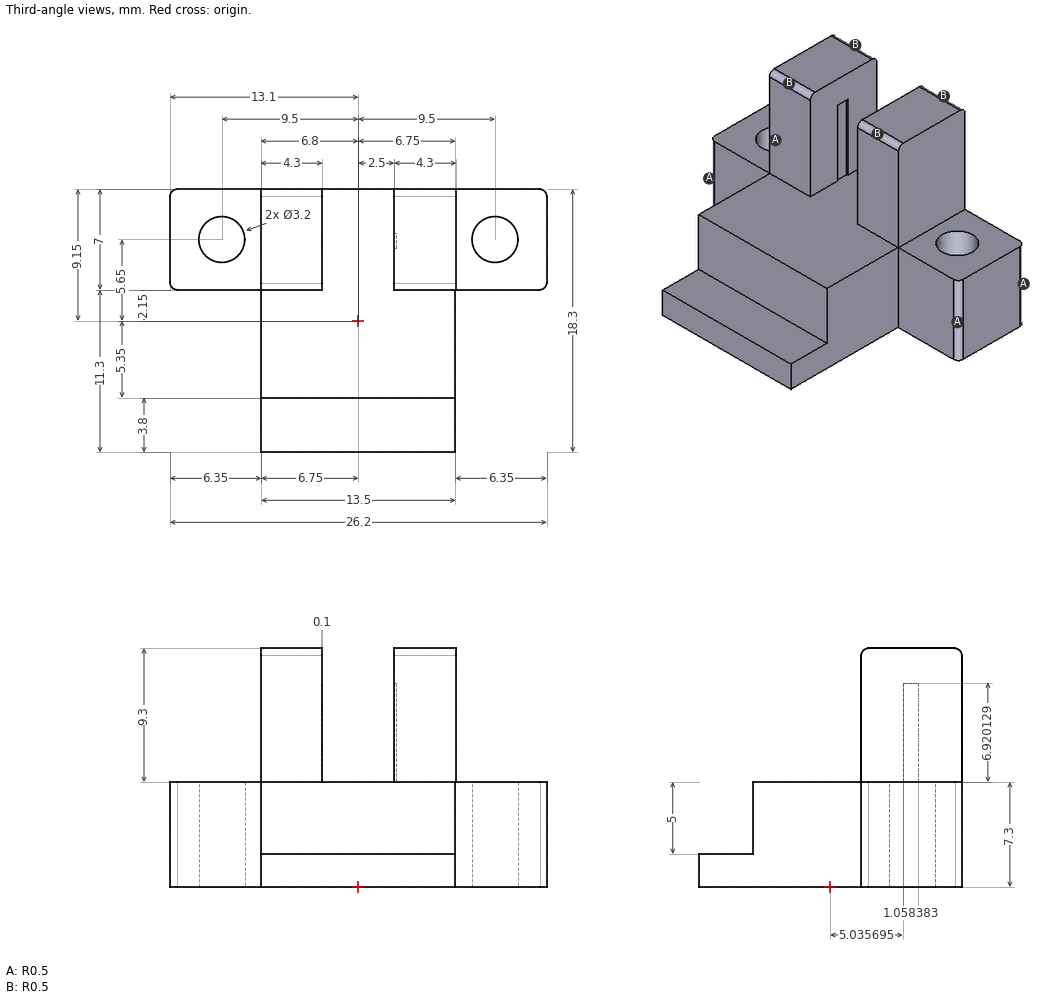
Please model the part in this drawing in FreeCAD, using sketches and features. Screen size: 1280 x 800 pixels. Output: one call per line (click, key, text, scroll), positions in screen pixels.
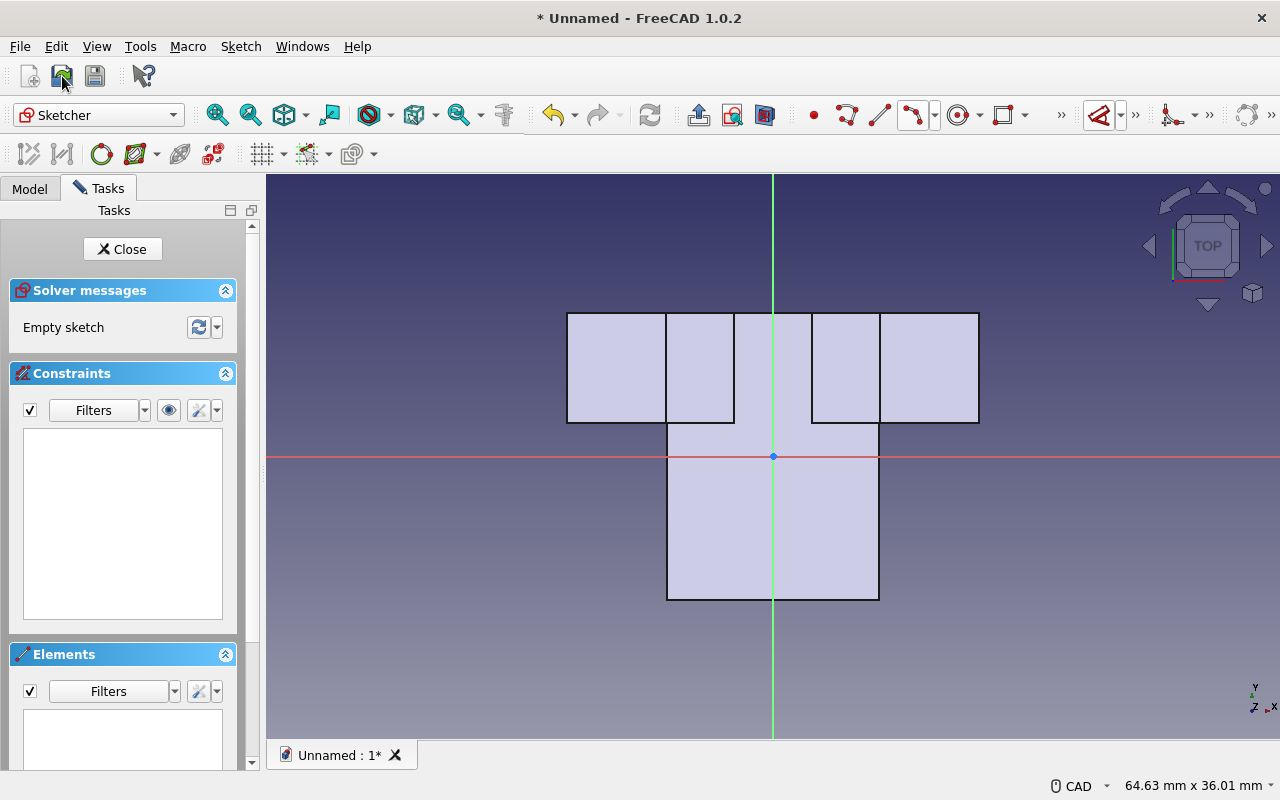
key(q)
key(s)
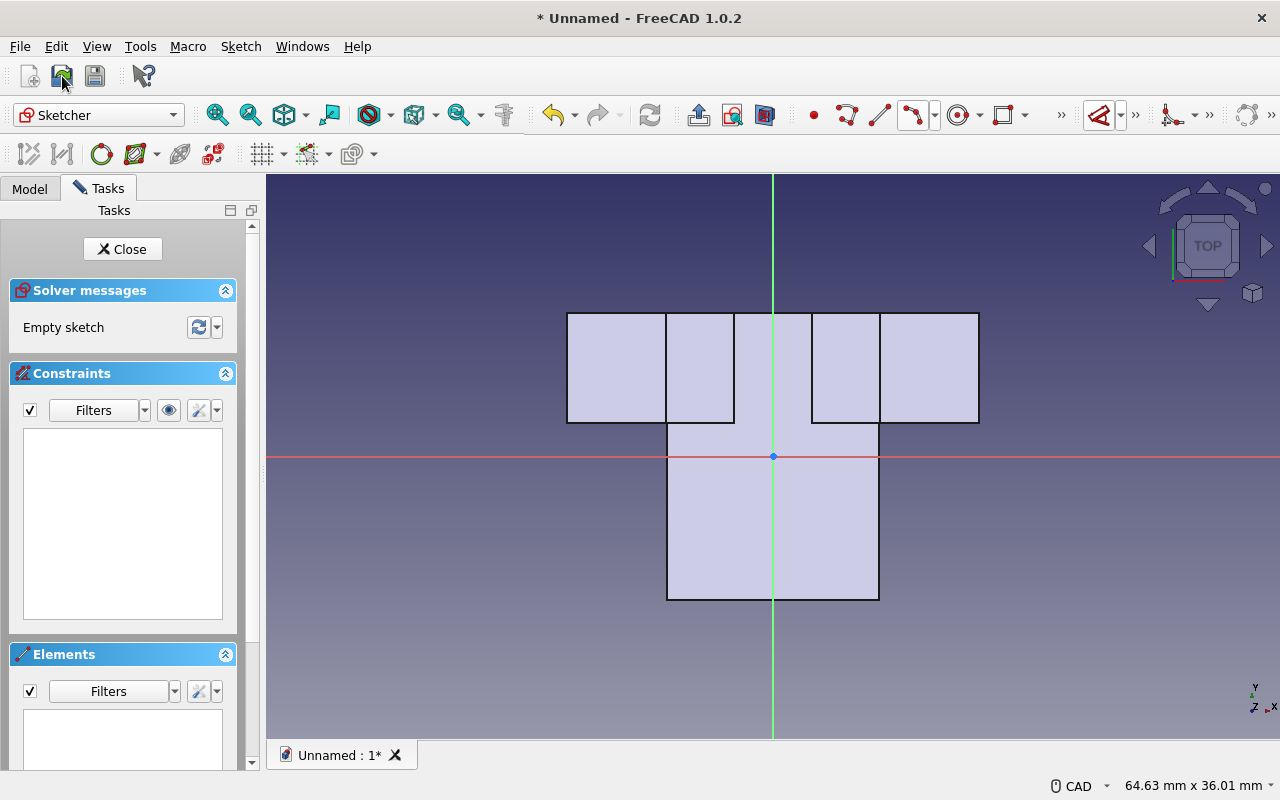
scroll(813, 570, up, 5)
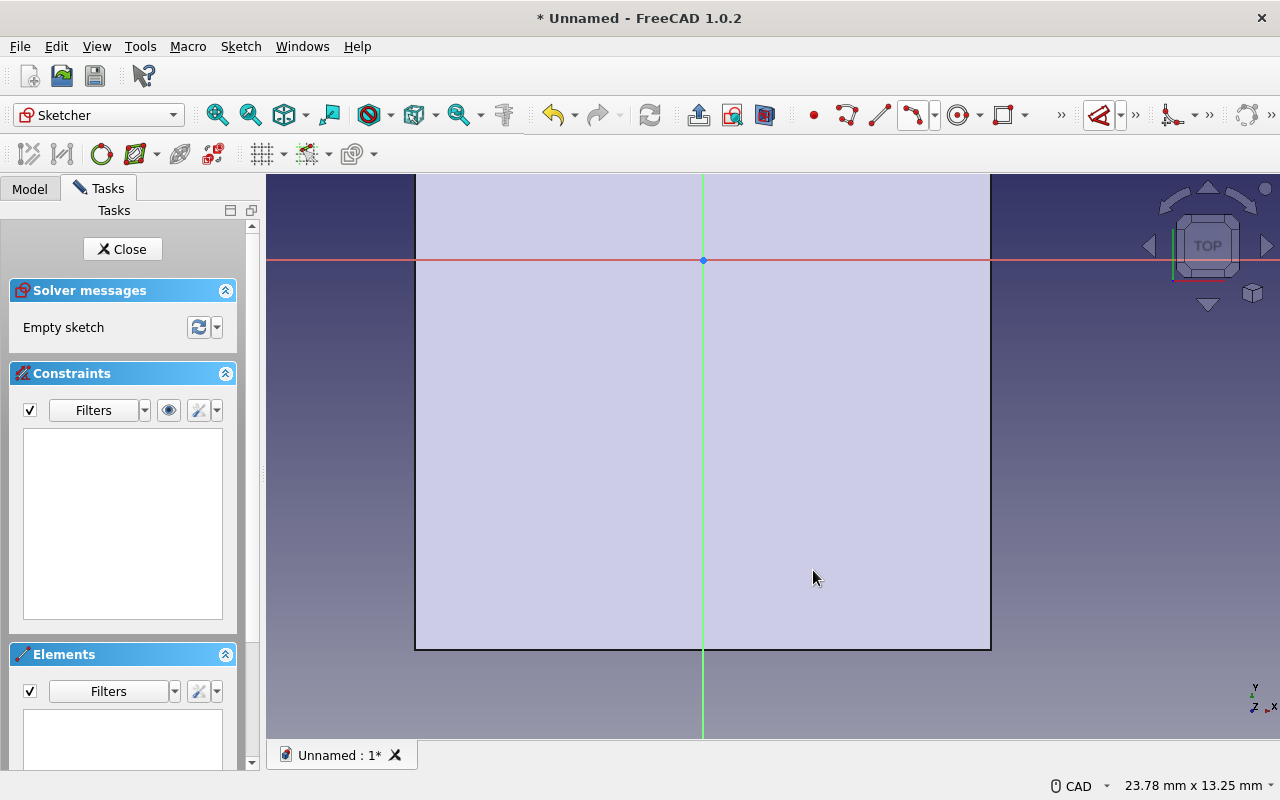
click(1002, 116)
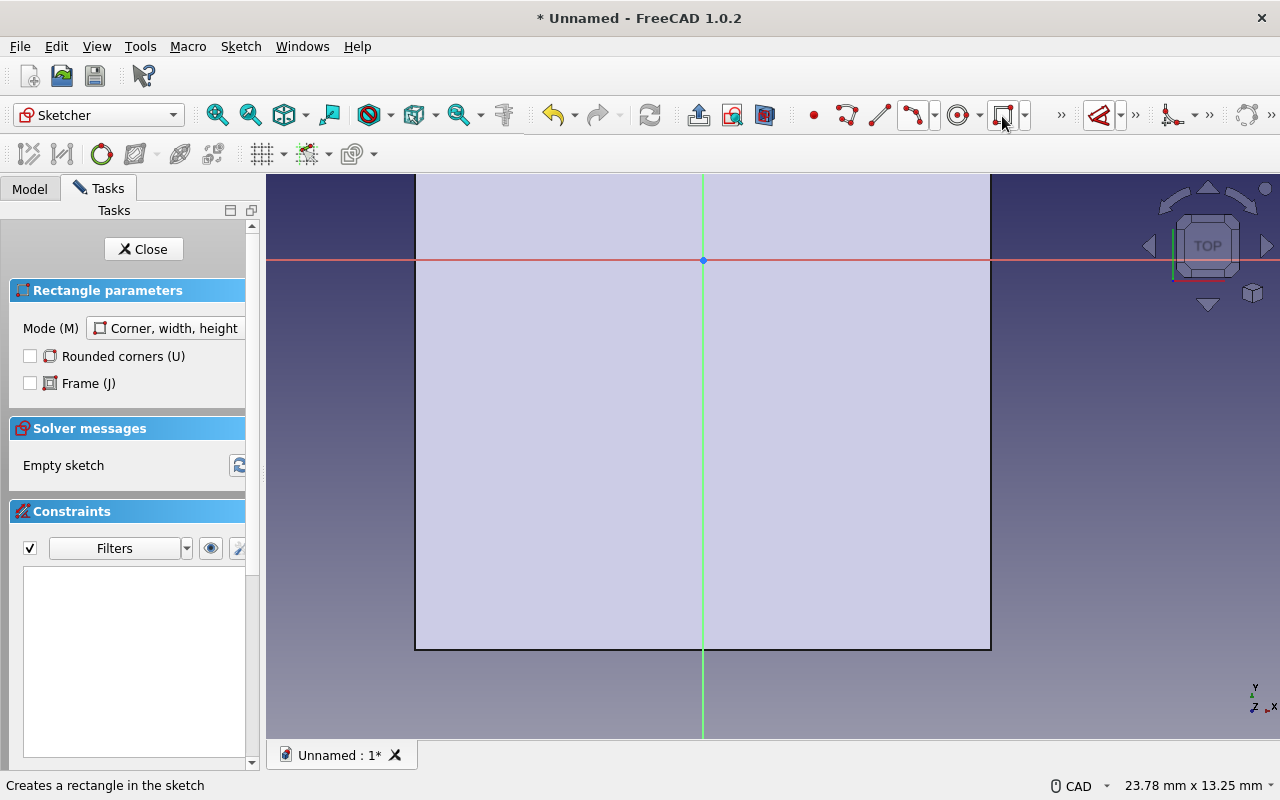
click(415, 488)
click(991, 650)
key(Escape)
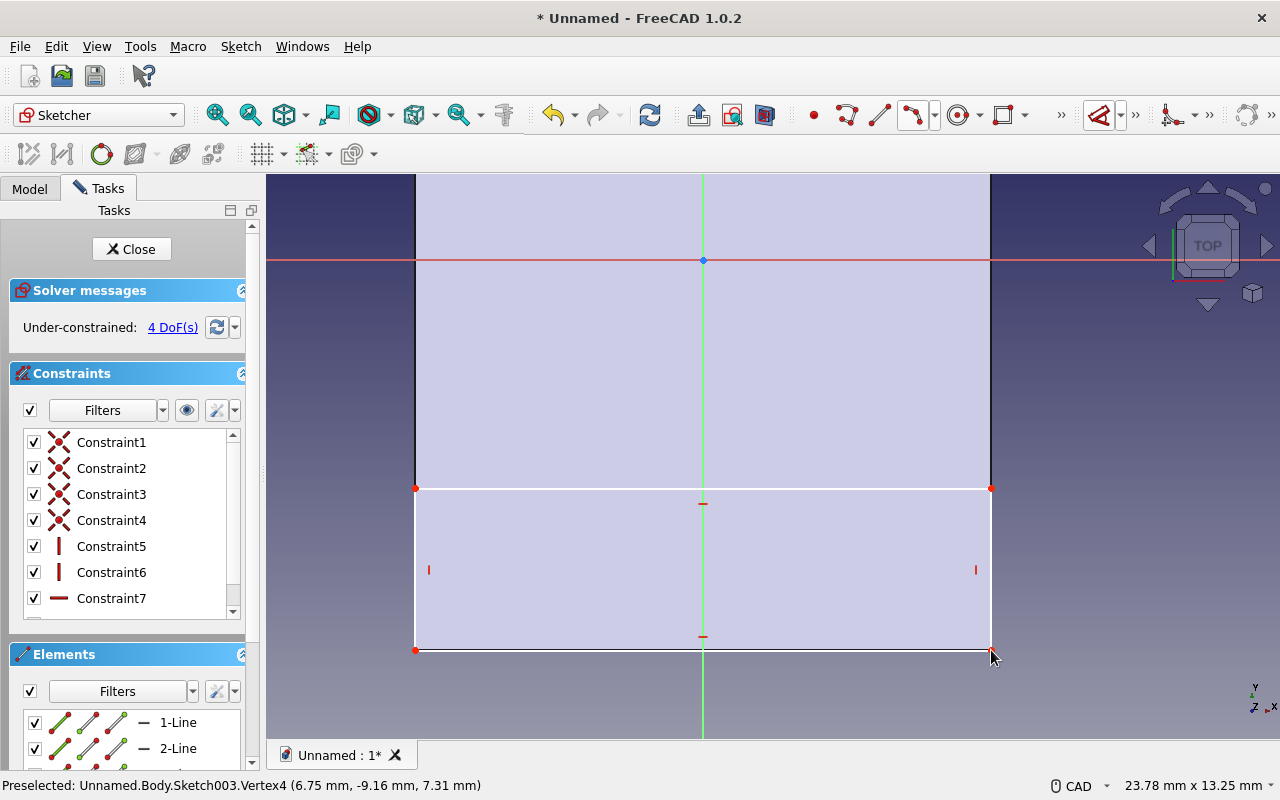
click(415, 538)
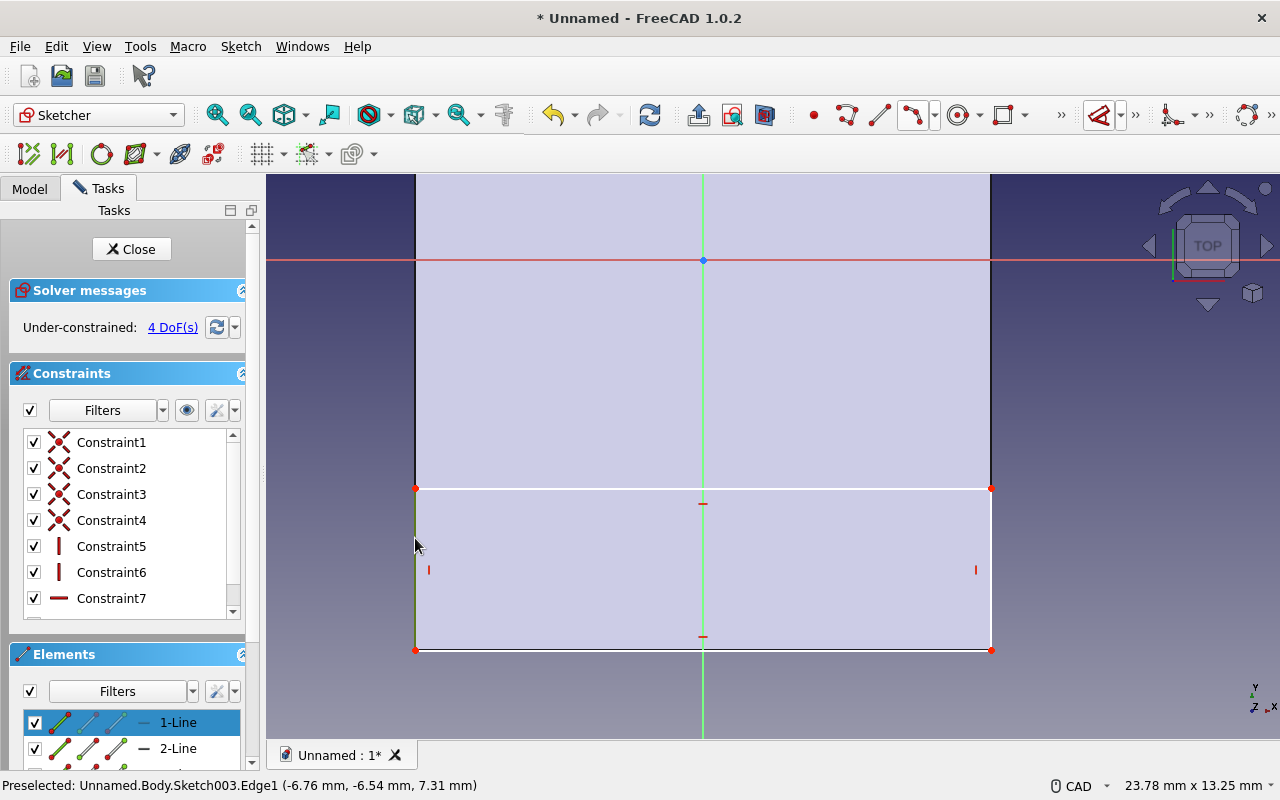
key(i)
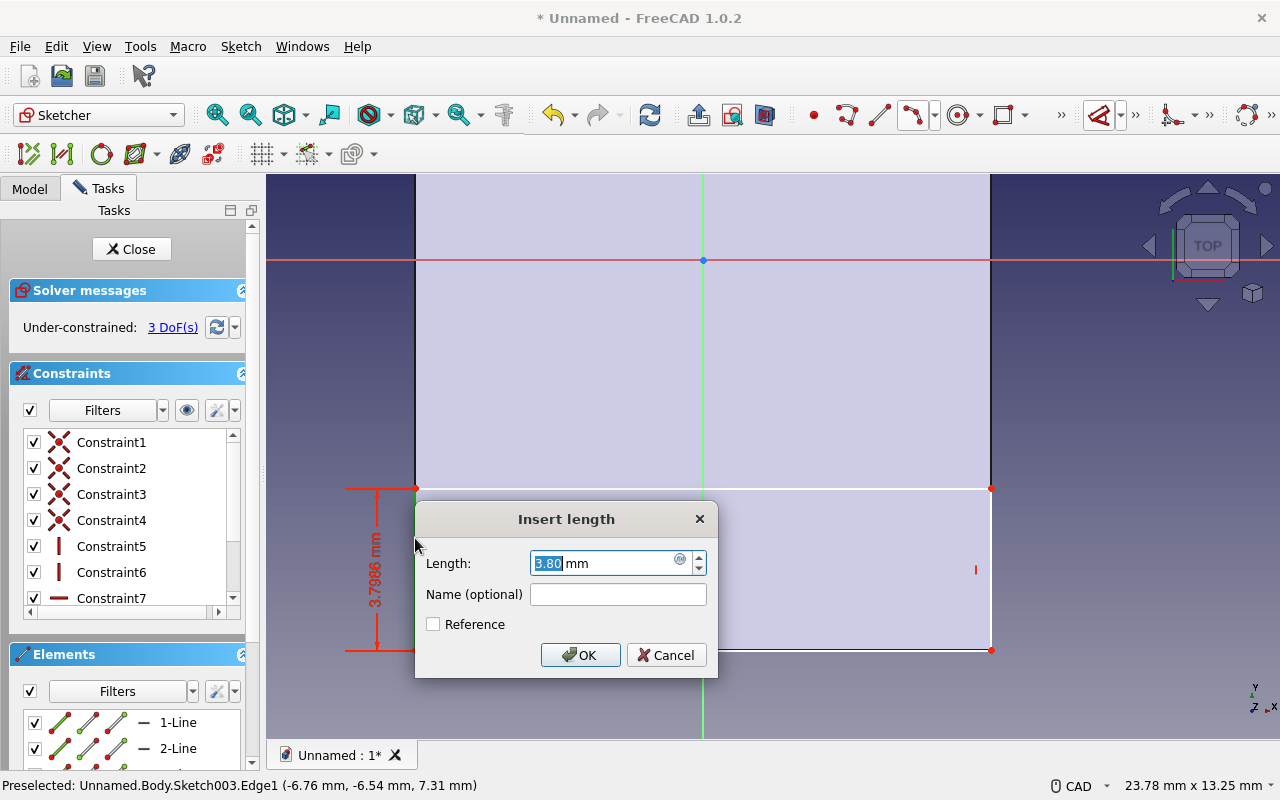
text(3.8)
key(Return)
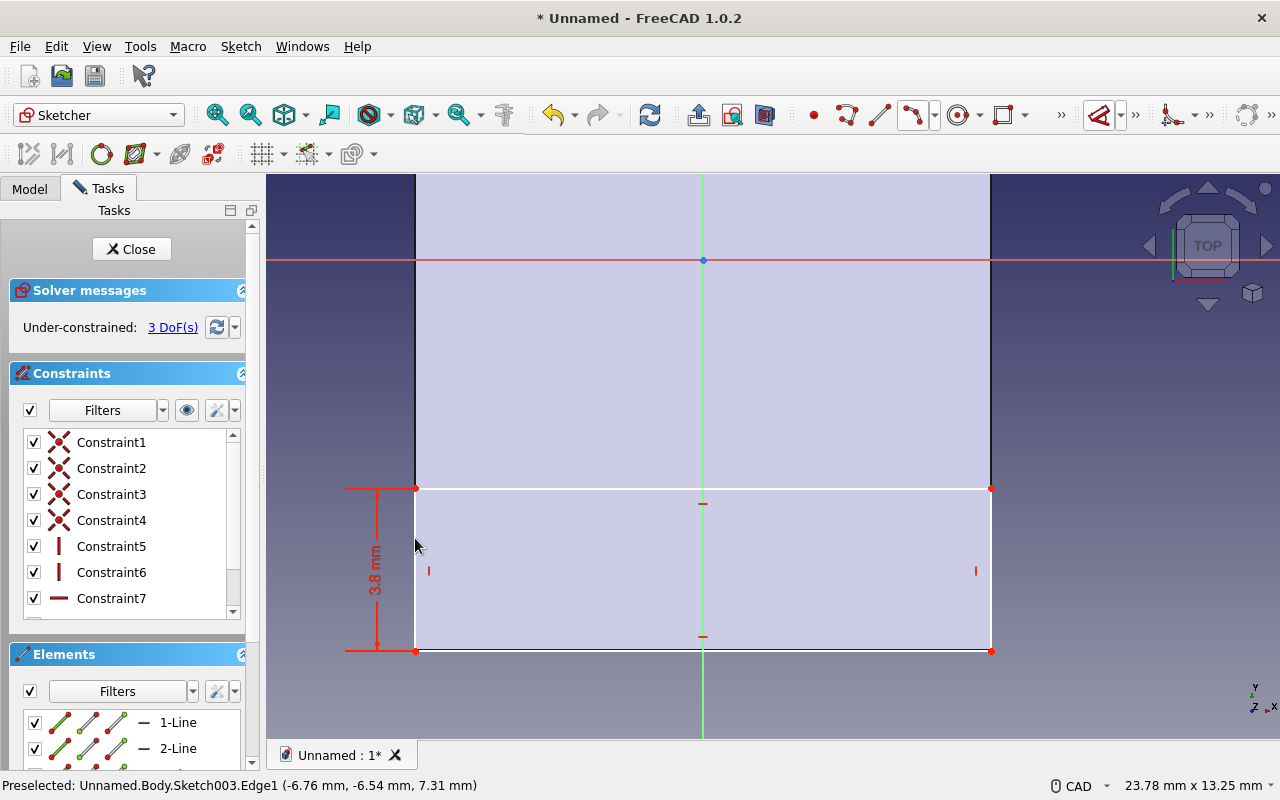
click(588, 651)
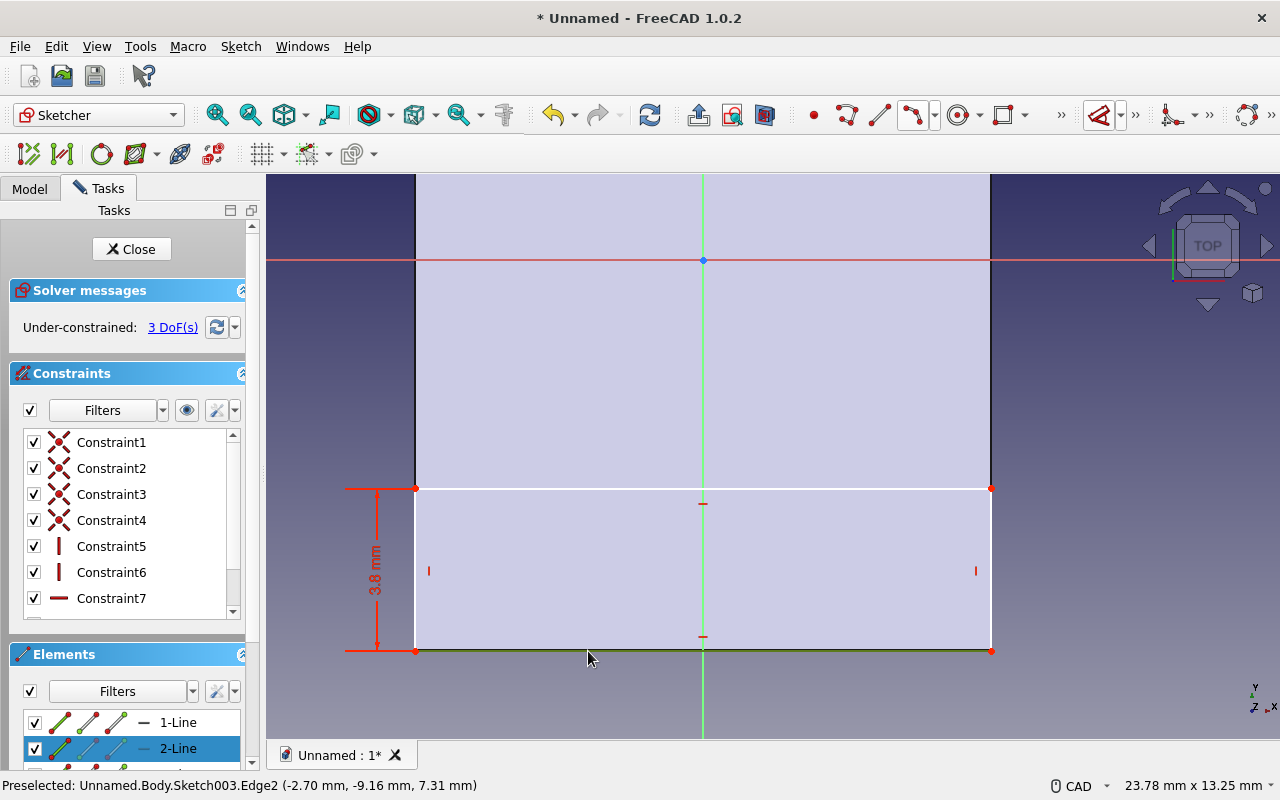
key(l)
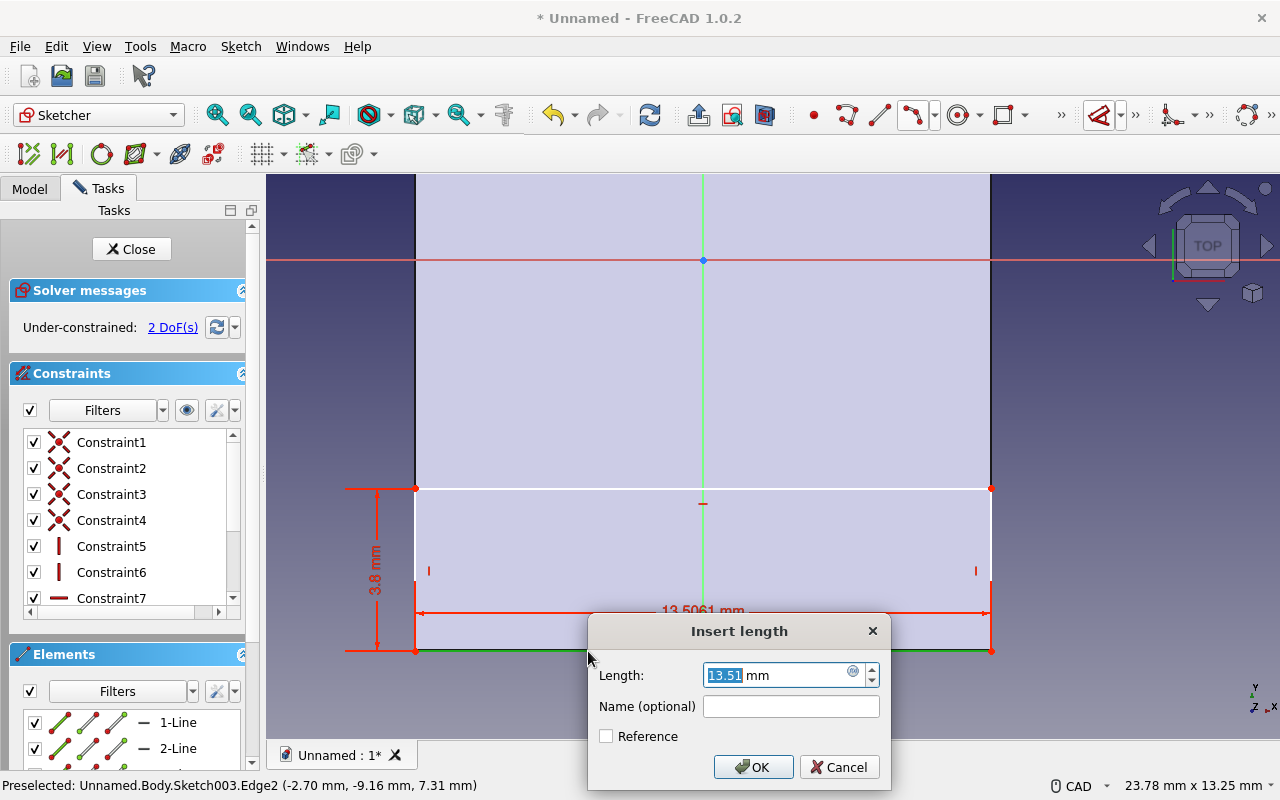
text(13.5)
key(Return)